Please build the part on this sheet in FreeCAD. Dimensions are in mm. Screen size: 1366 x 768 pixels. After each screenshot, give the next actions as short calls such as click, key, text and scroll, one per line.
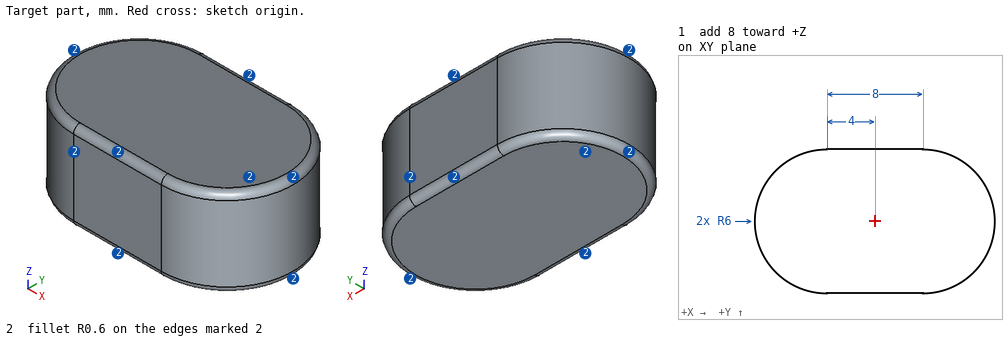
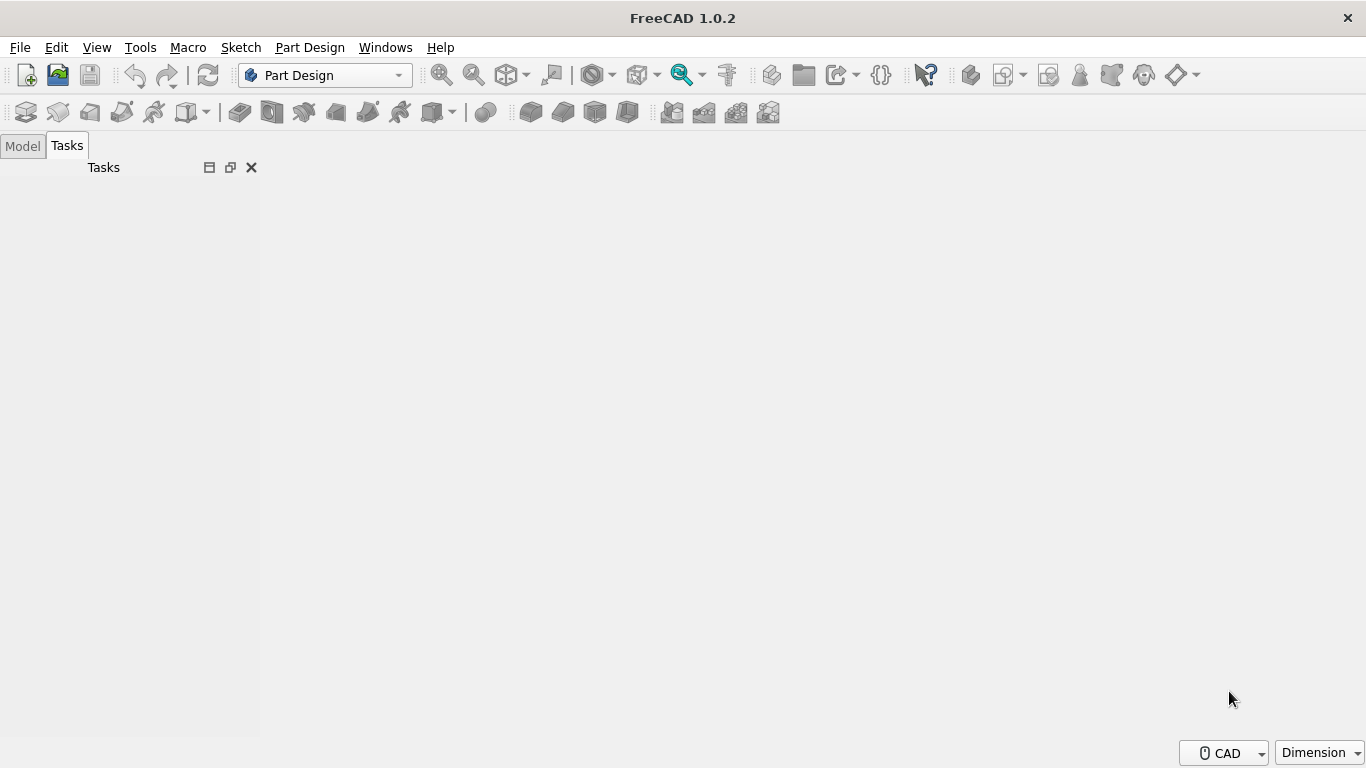
key(ctrl+n)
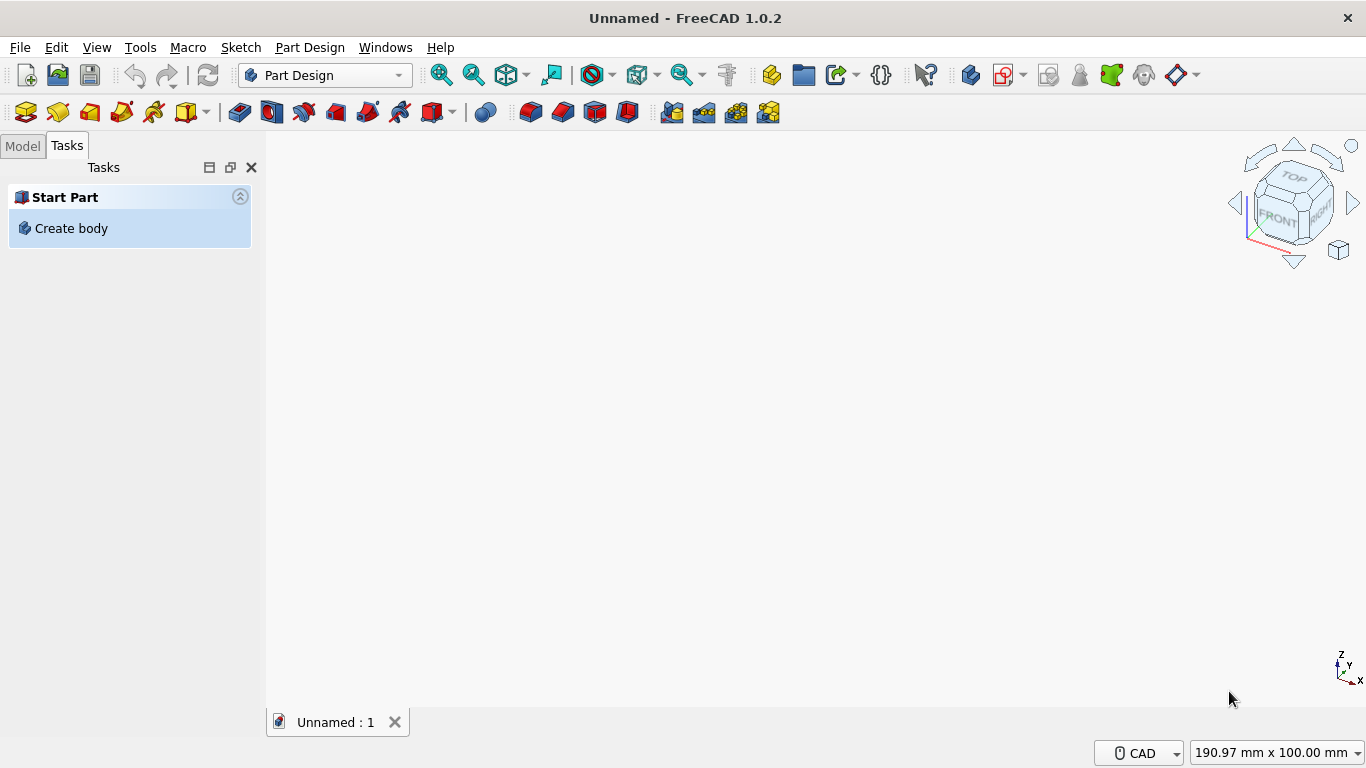
click(1004, 76)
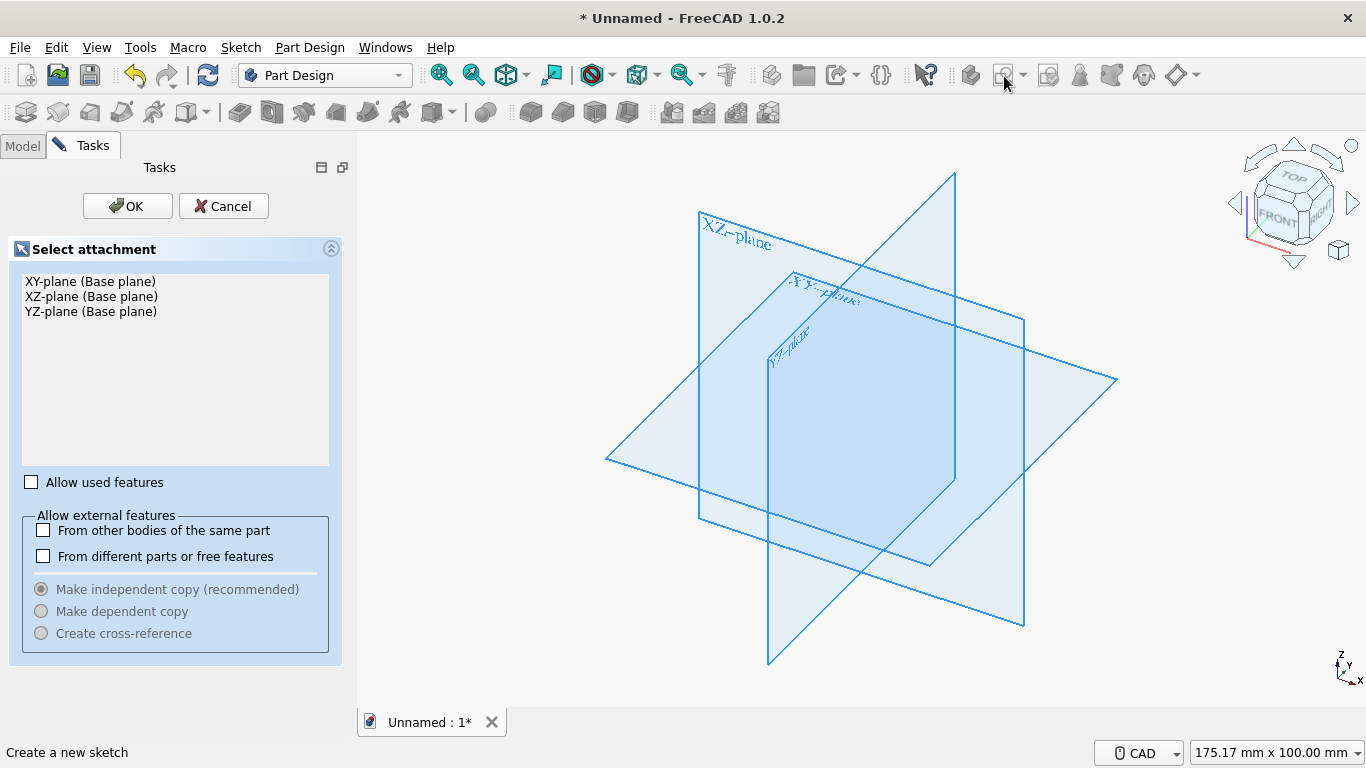
click(82, 282)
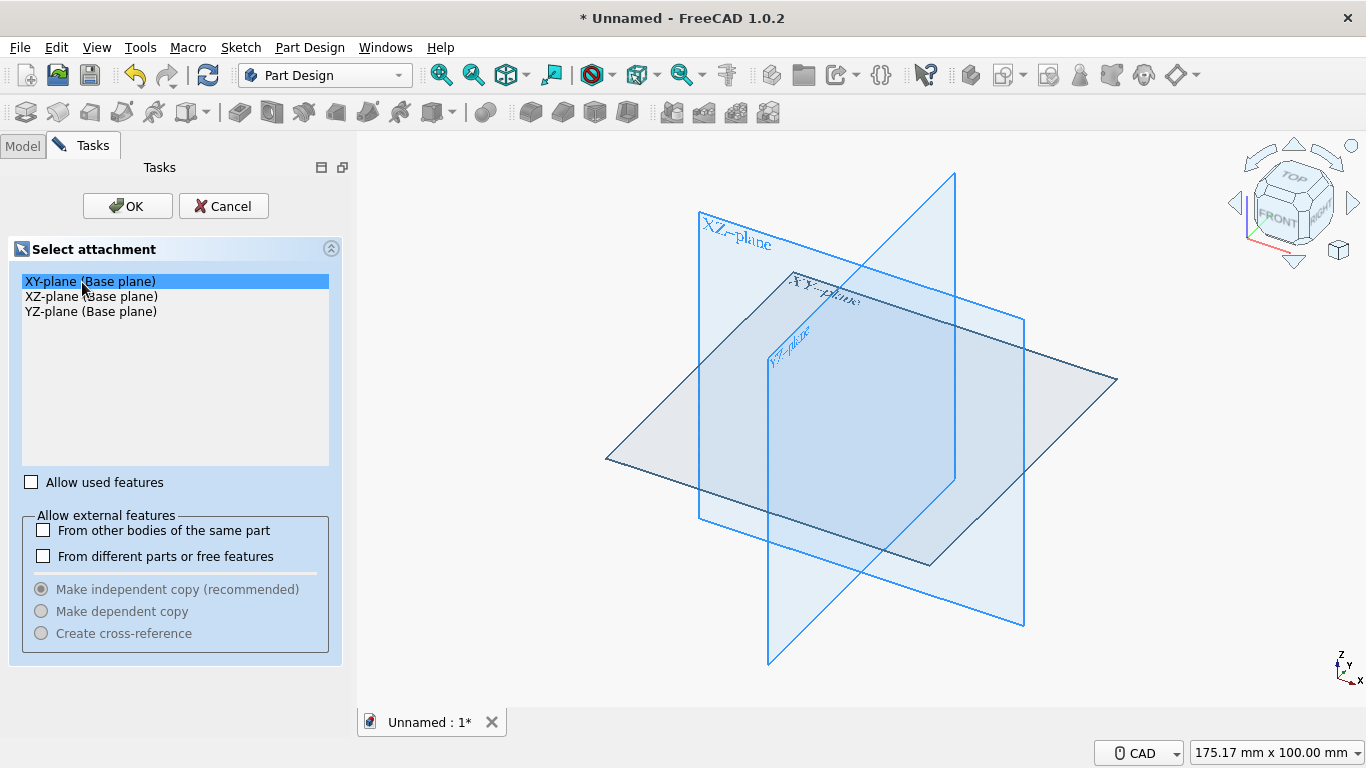
click(128, 206)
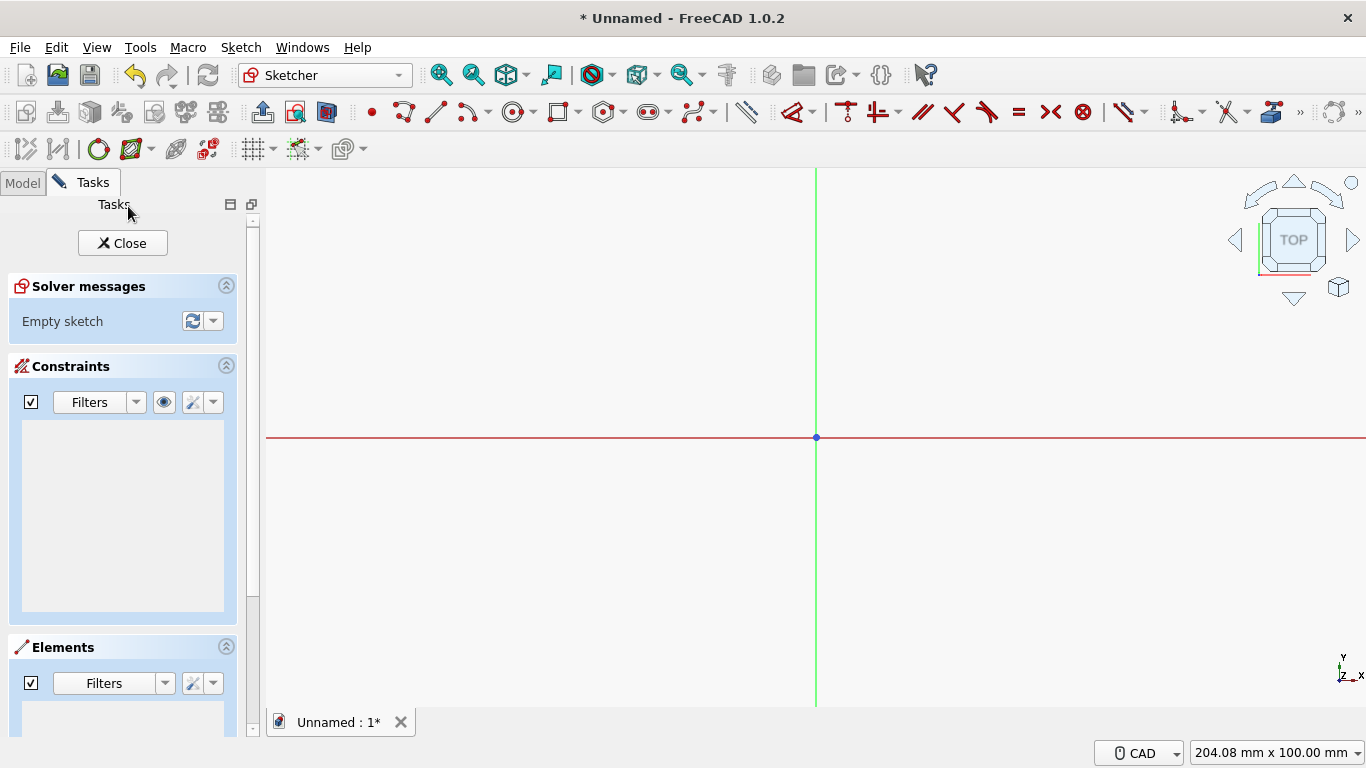
scroll(833, 438, up, 8)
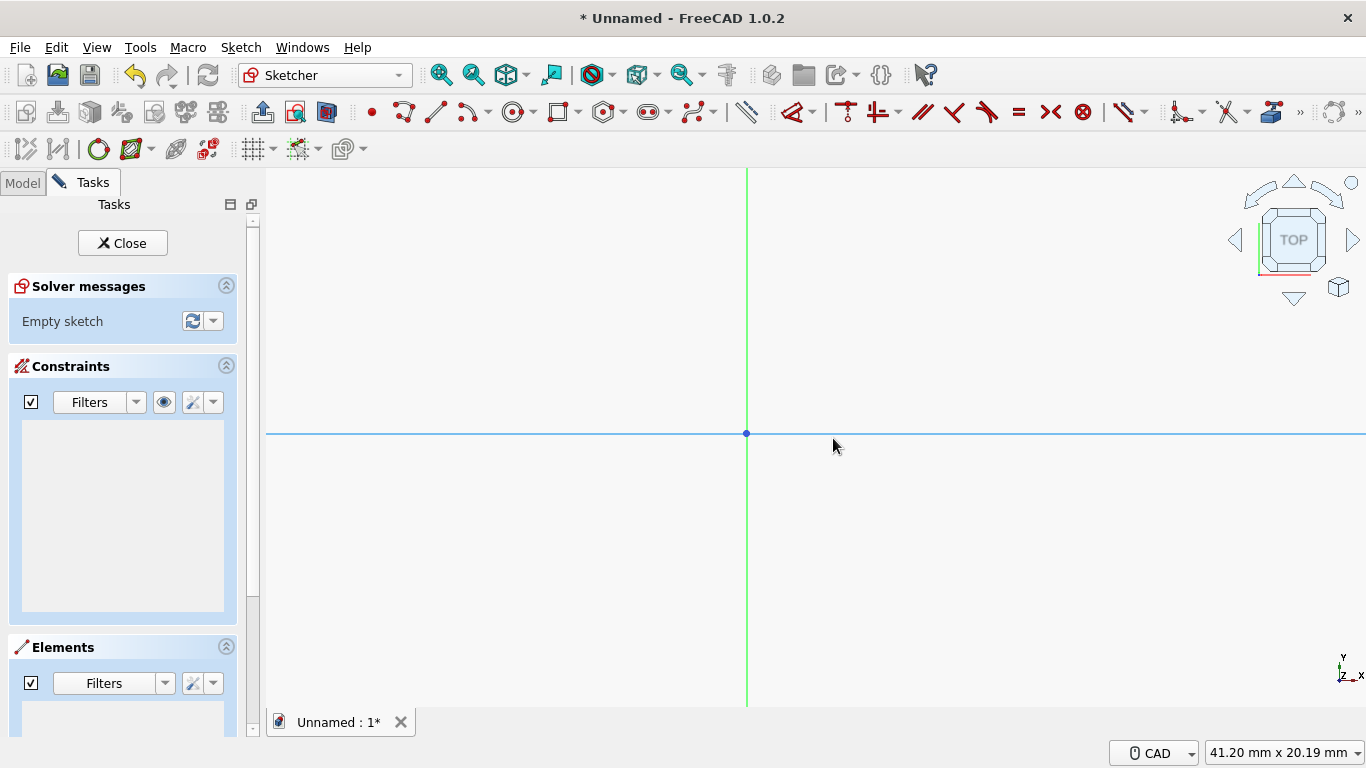
key(g)
key(s)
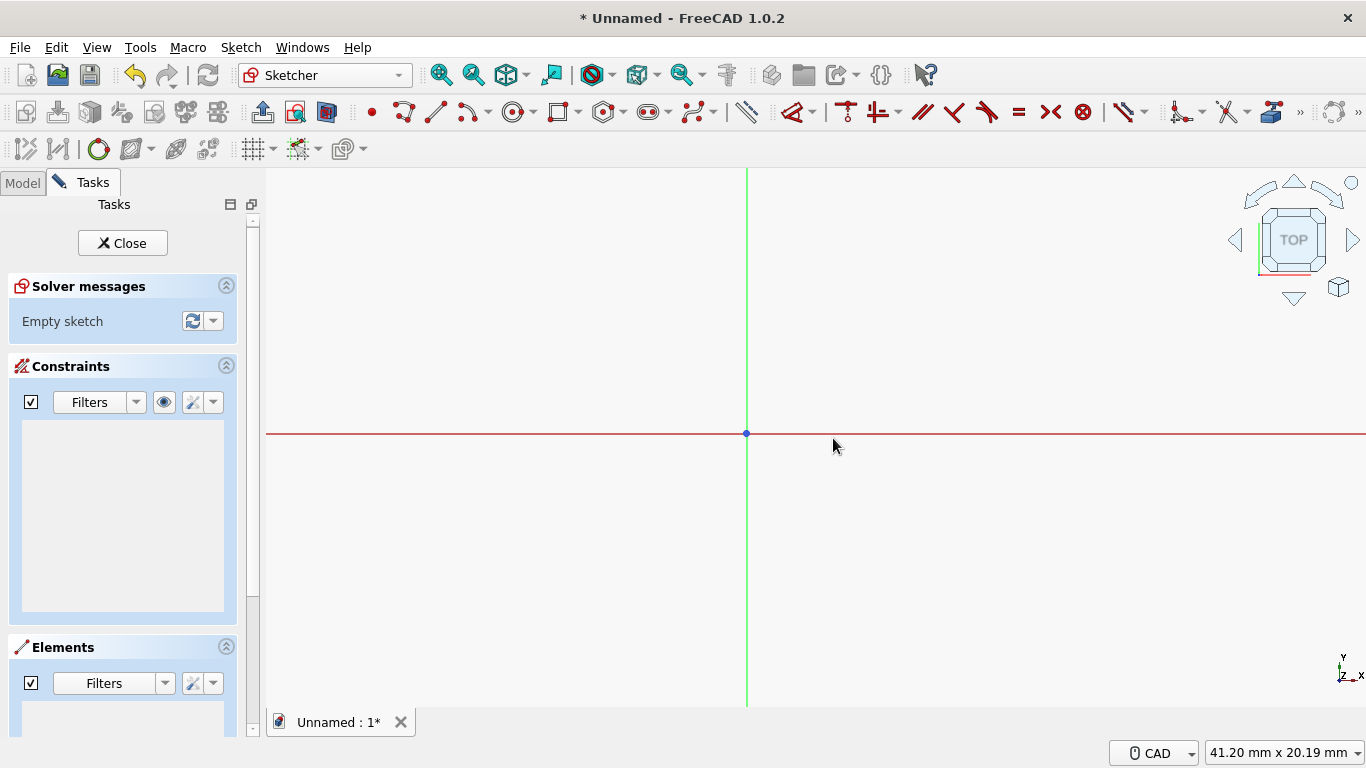
click(640, 434)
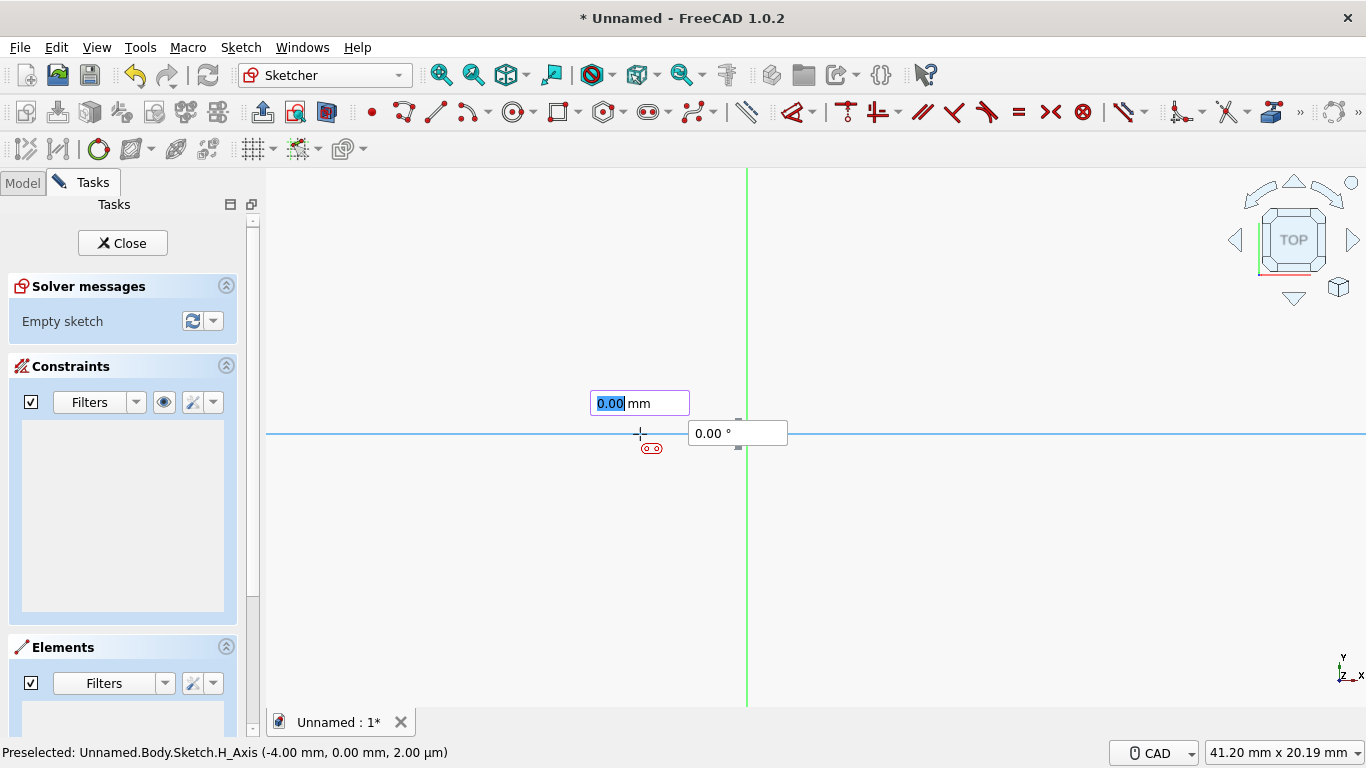
click(854, 425)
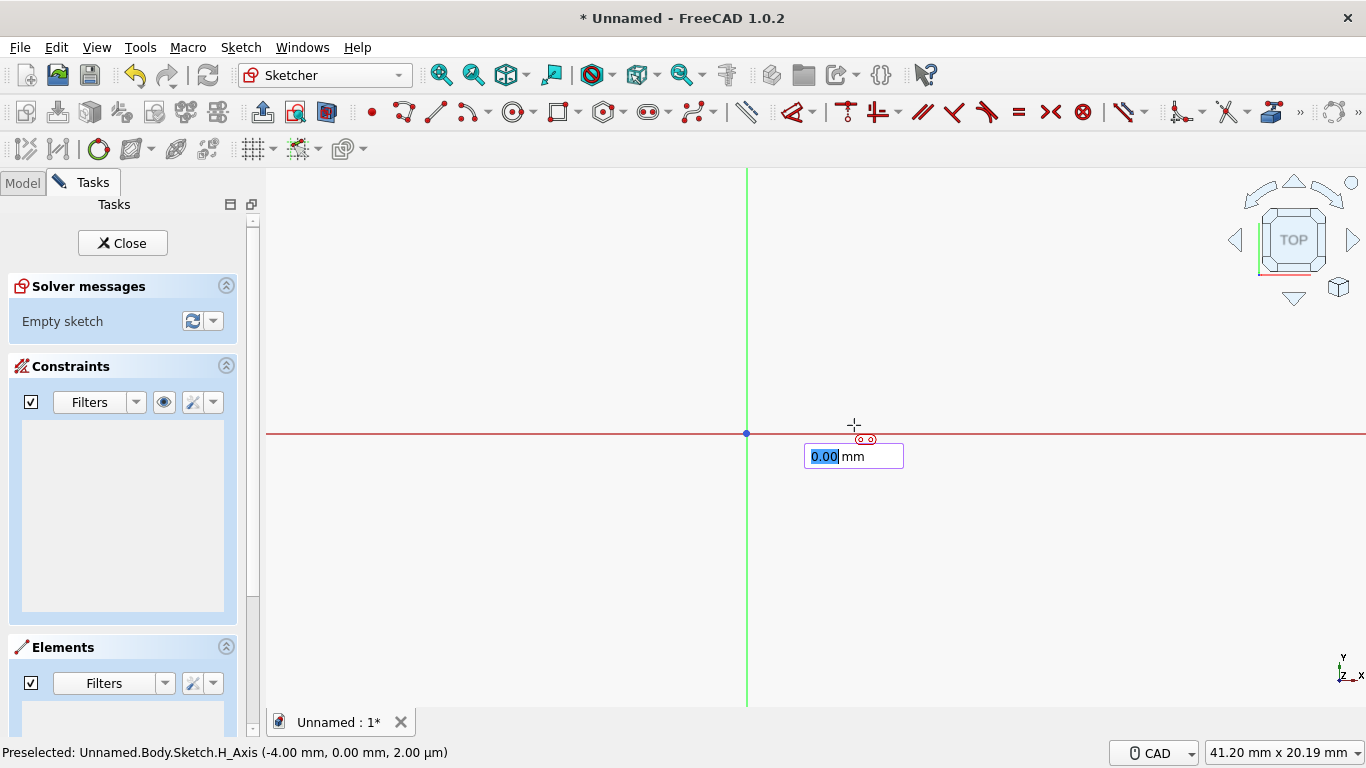
click(779, 273)
key(Escape)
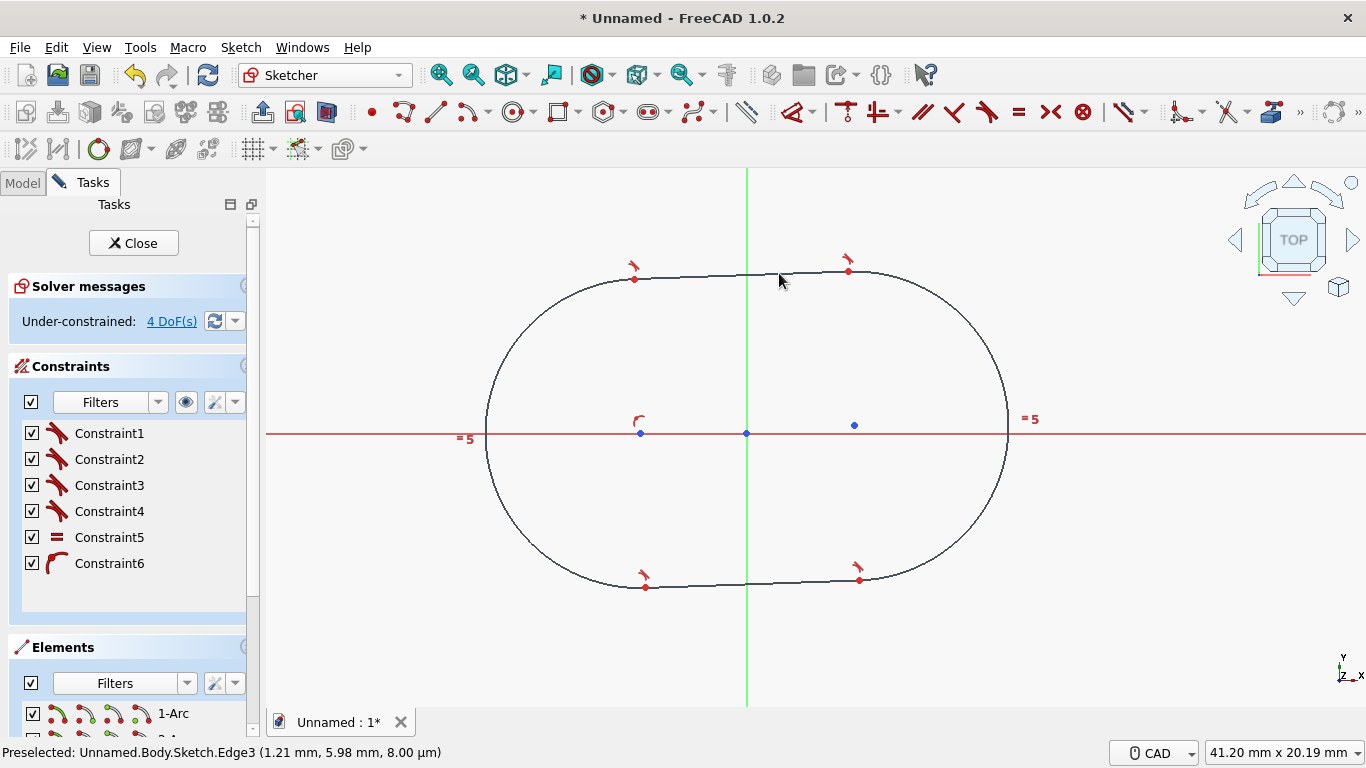
click(699, 277)